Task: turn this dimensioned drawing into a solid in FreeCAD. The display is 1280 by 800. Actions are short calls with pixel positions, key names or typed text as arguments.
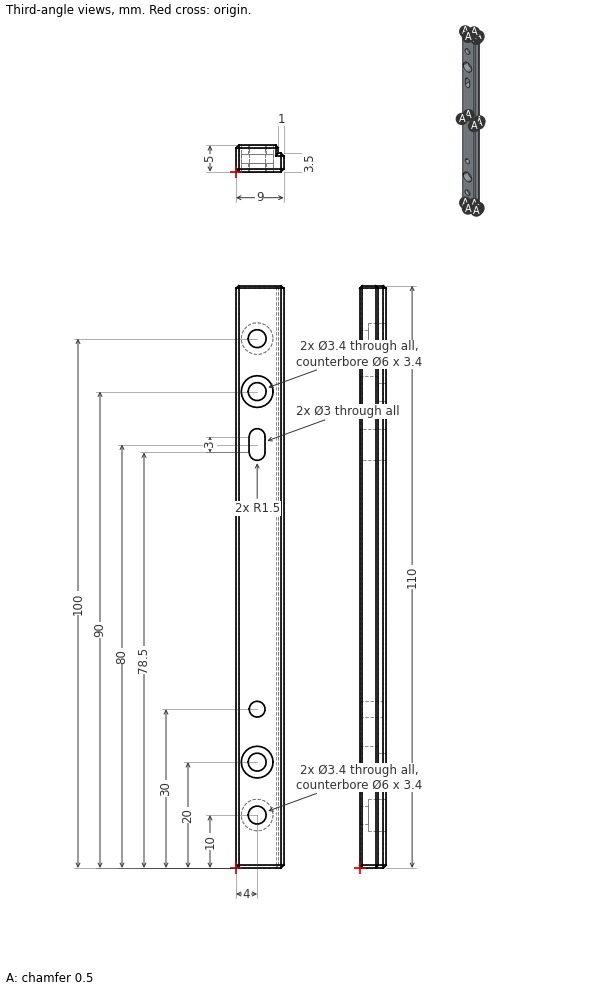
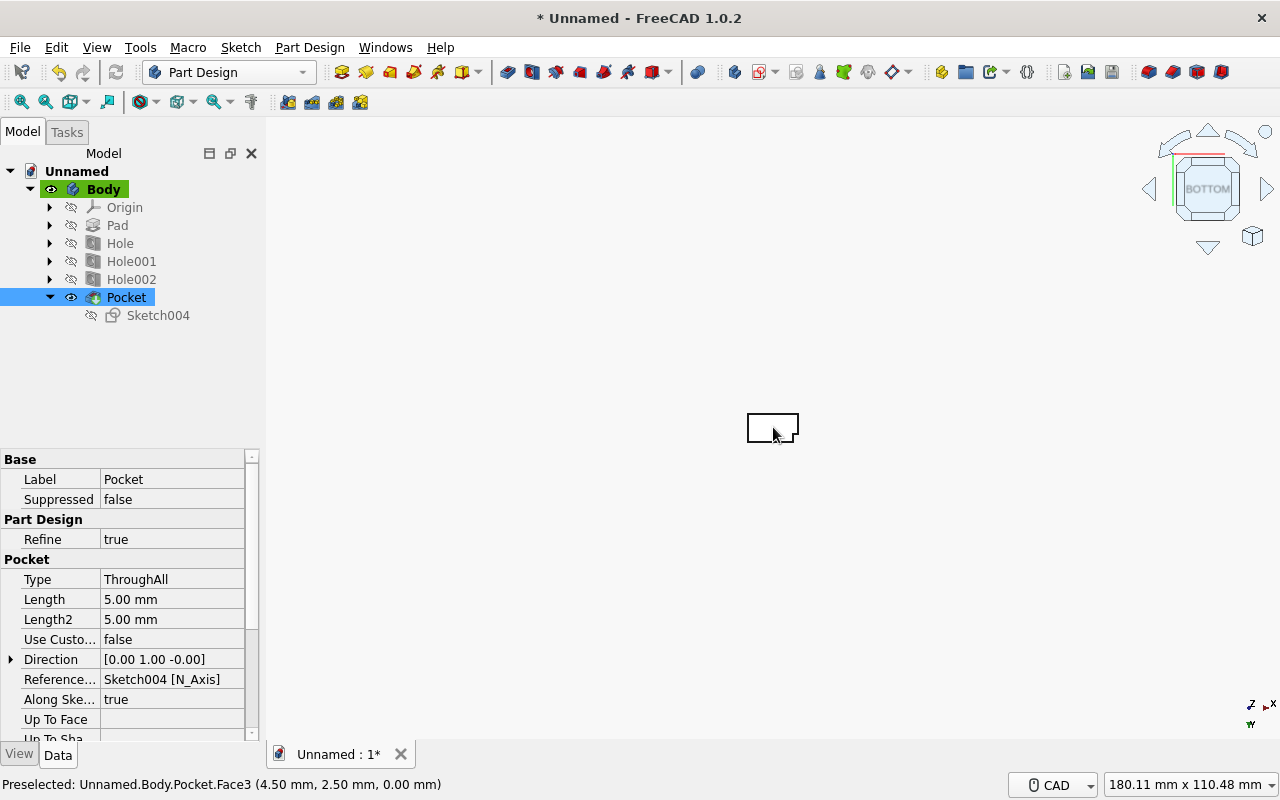
key(4)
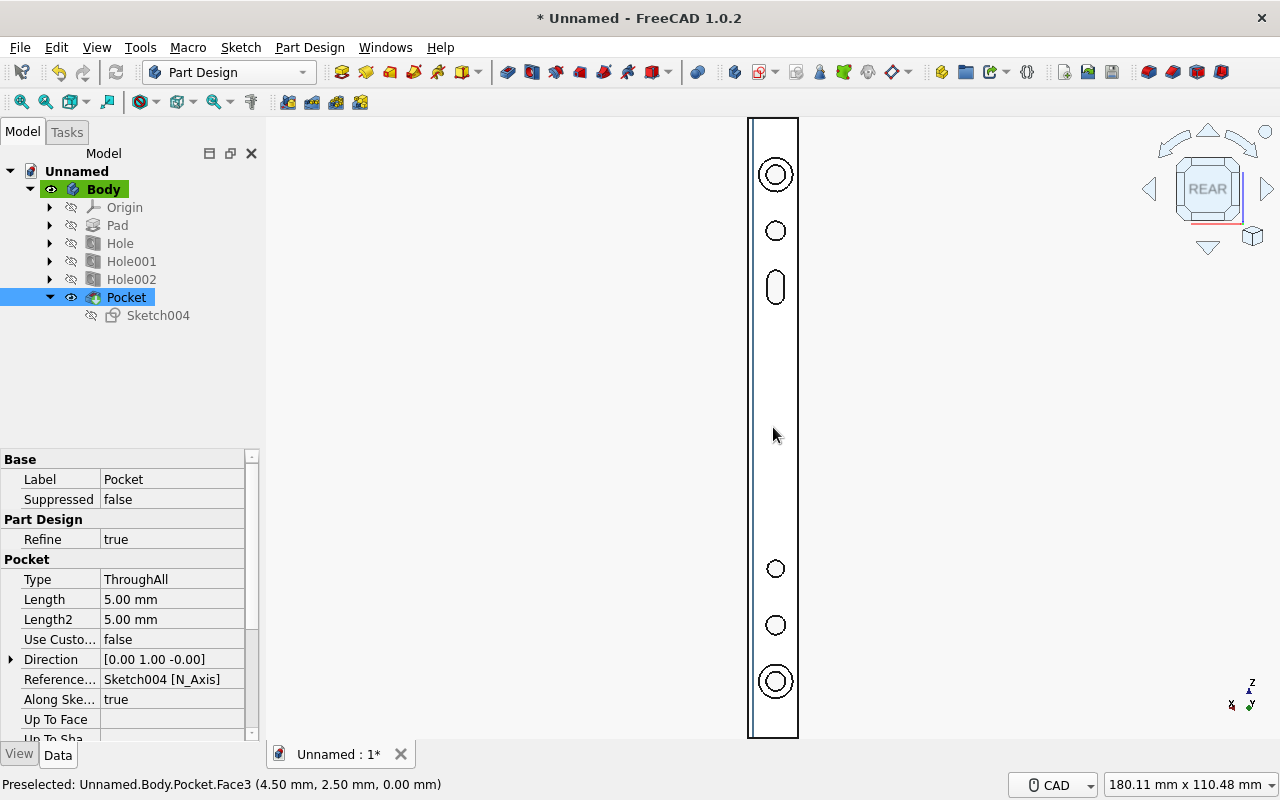
key(6)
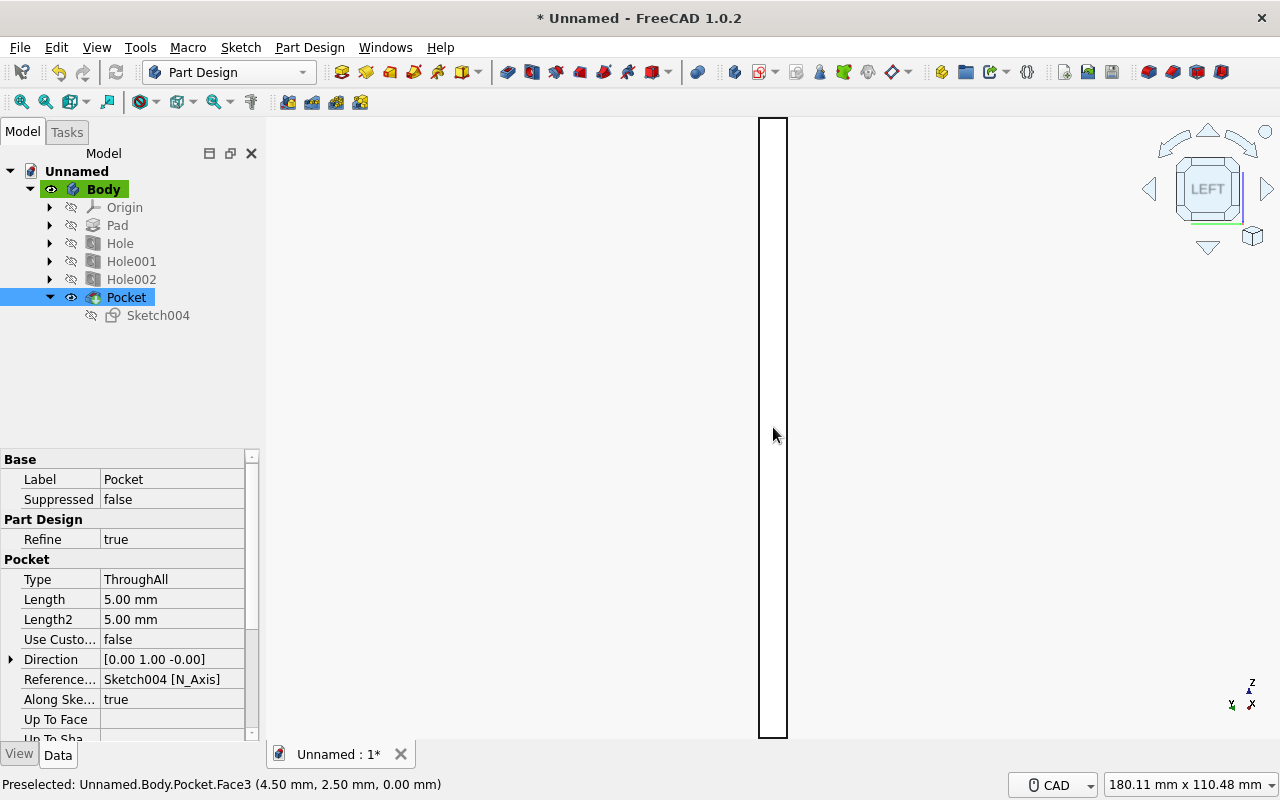
click(773, 162, ctrl)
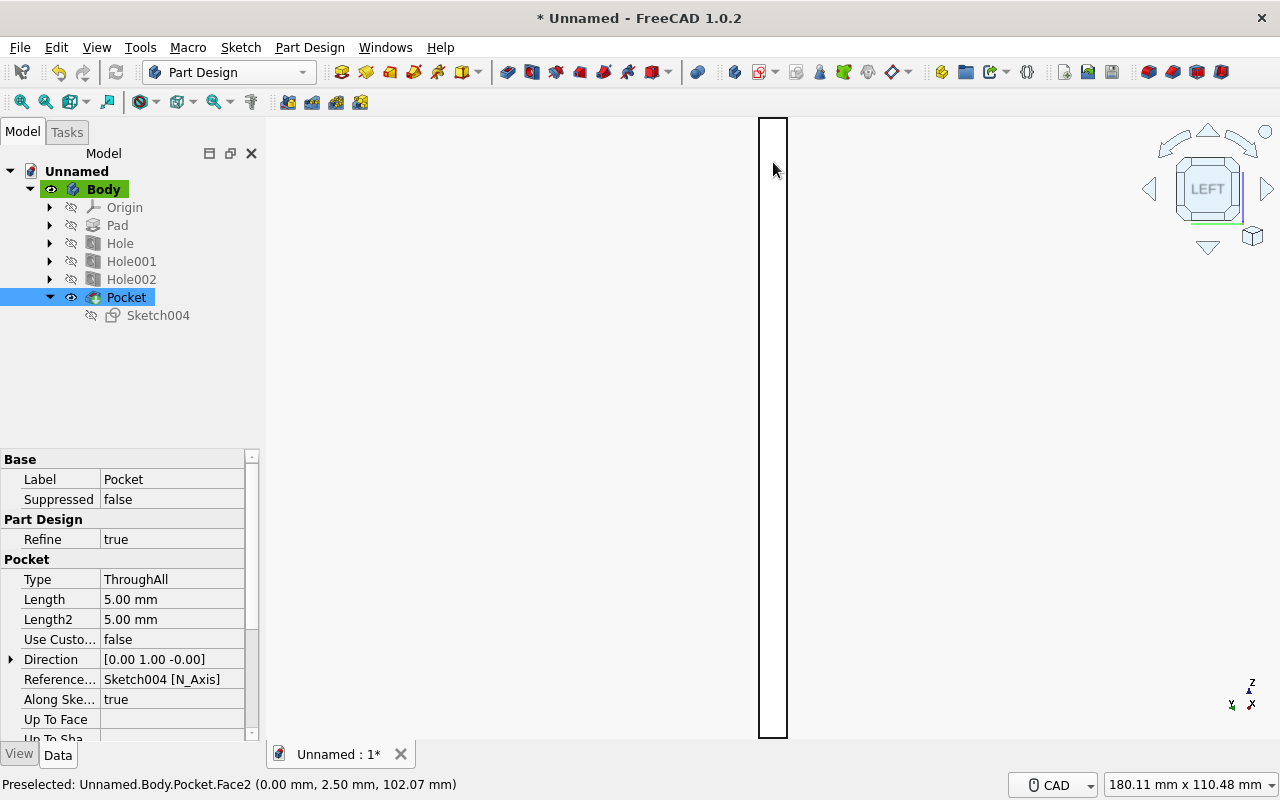
click(1174, 72)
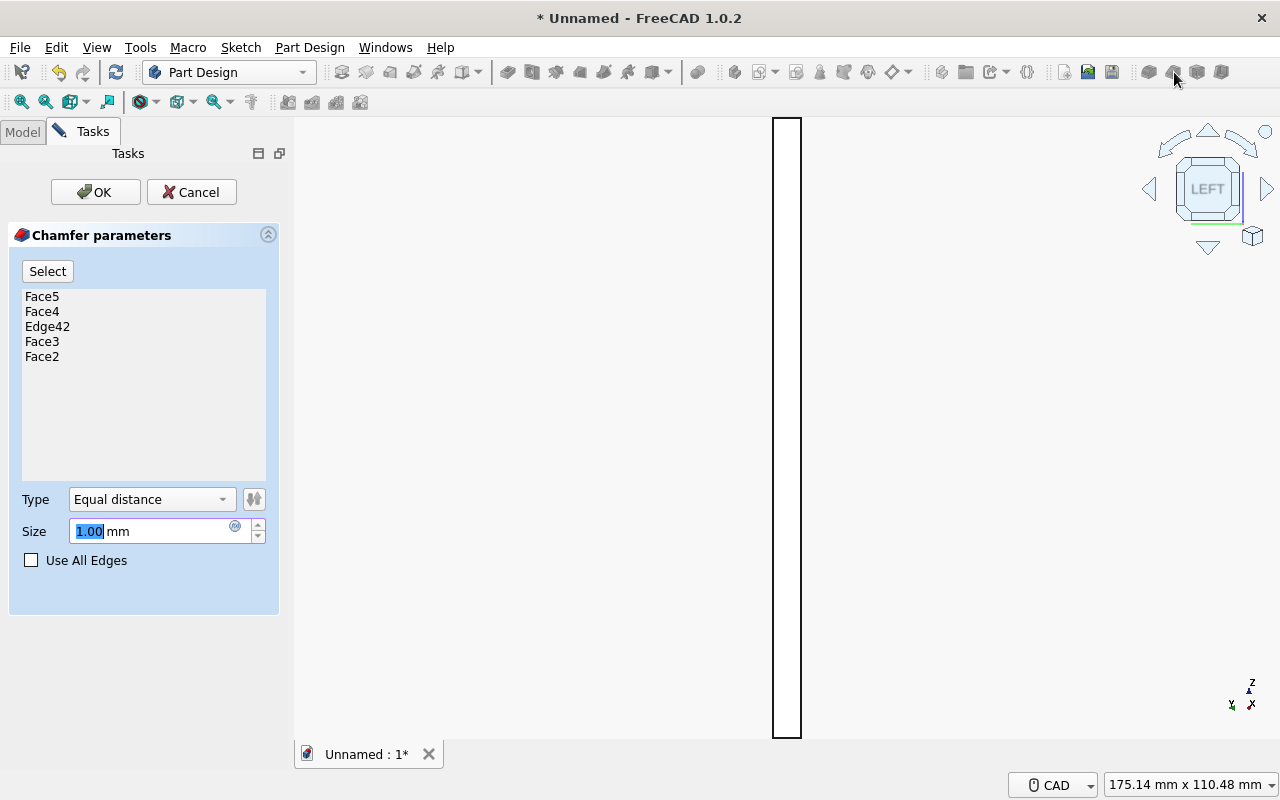
text(0.5)
key(Tab)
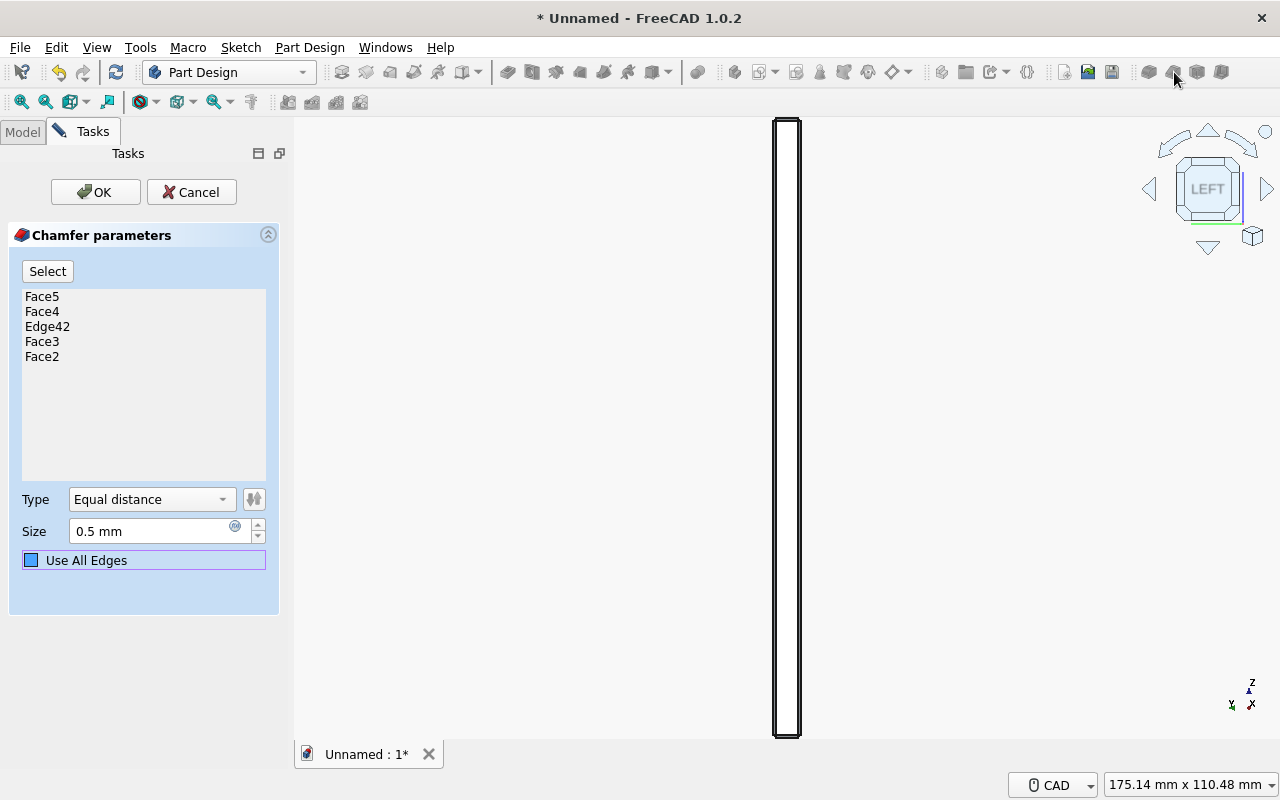
click(96, 192)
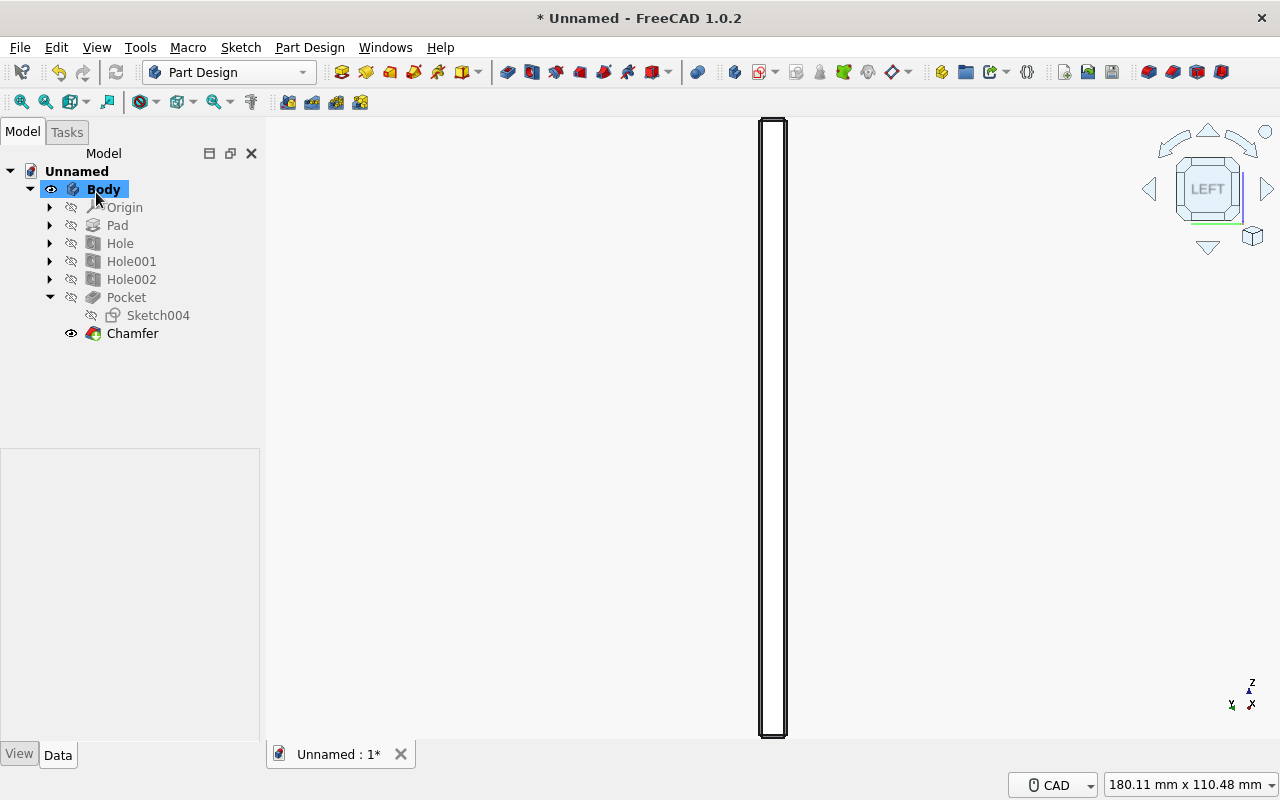
key(0)